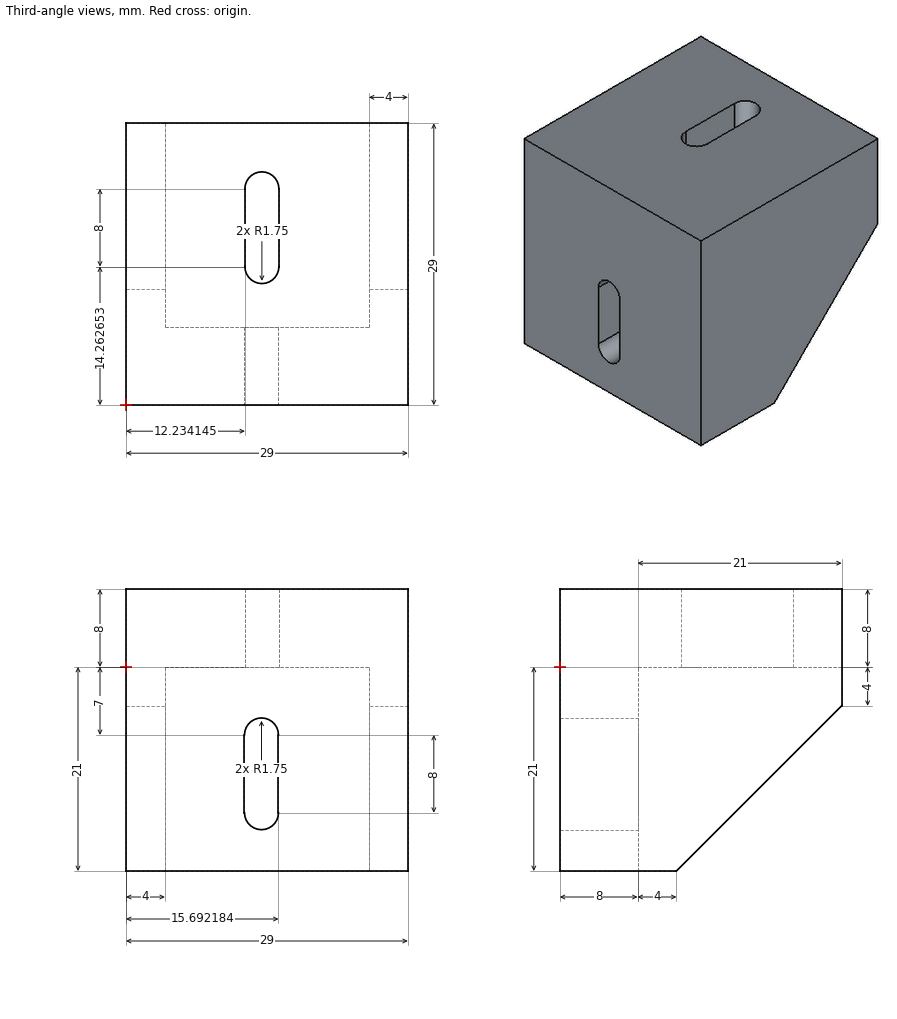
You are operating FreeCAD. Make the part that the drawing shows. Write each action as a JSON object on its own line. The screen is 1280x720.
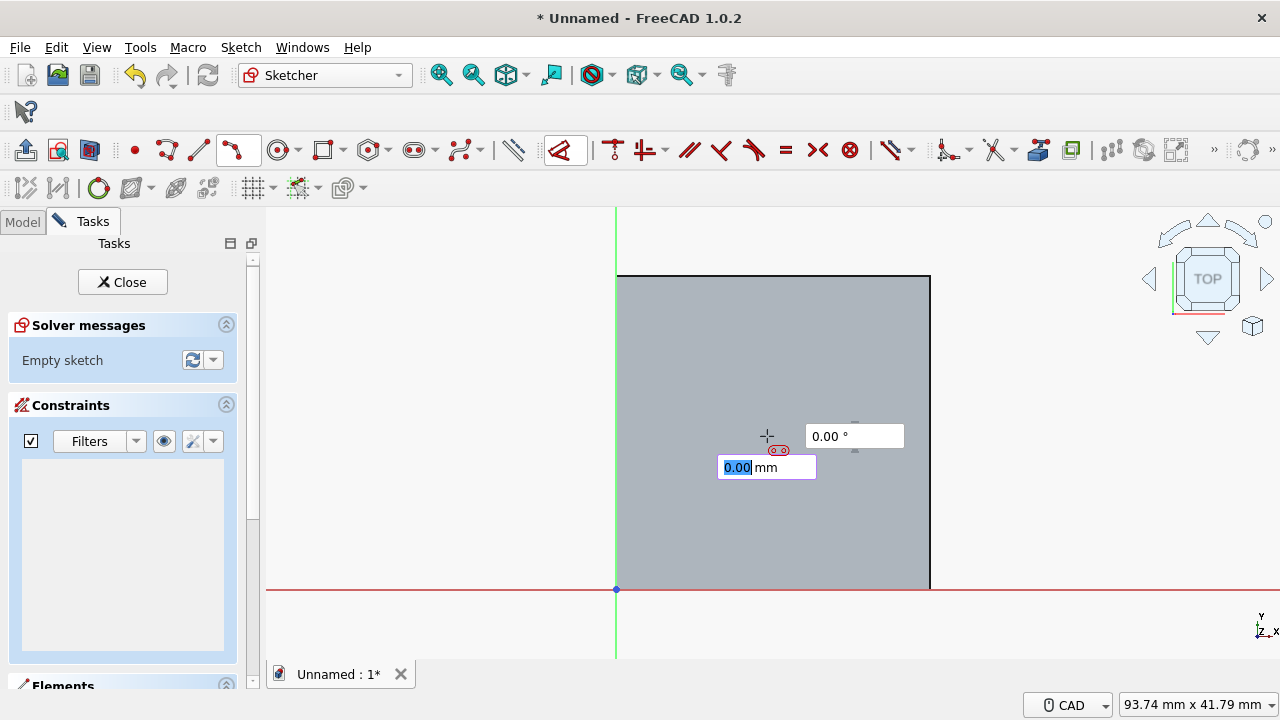
{"action": "left_click", "coordinate": [767, 349]}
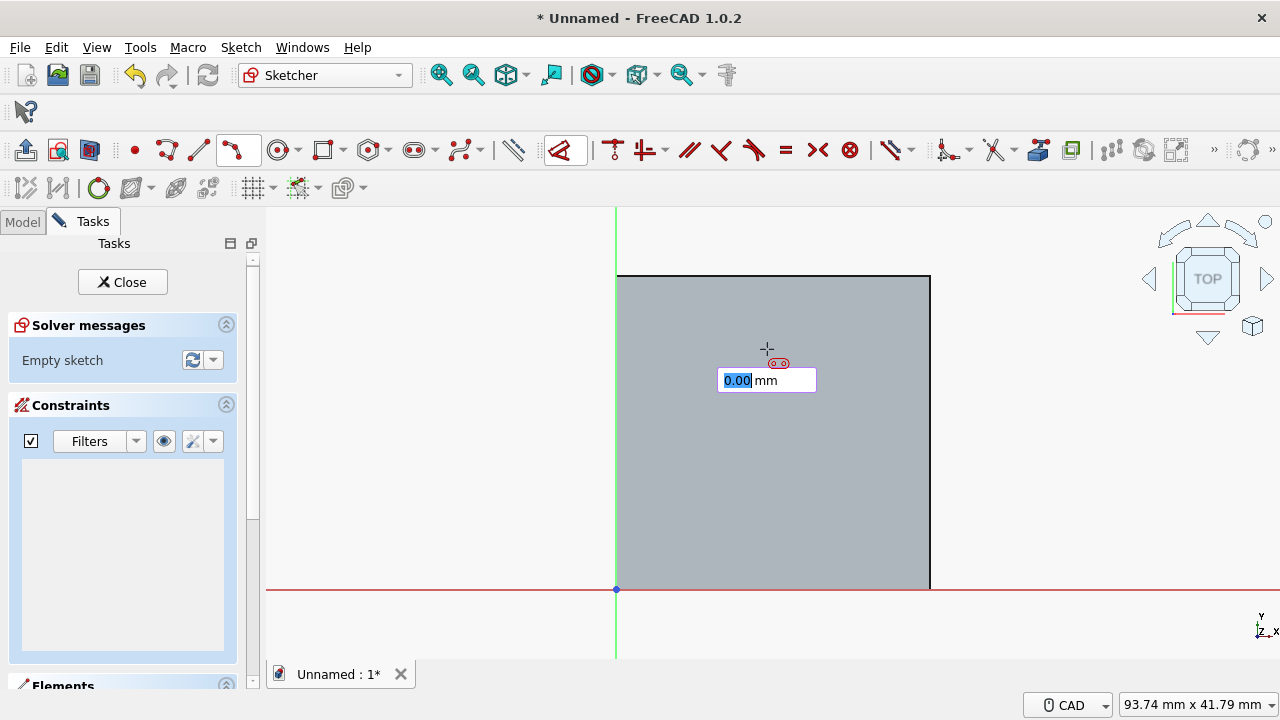
{"action": "left_click", "coordinate": [748, 392]}
{"action": "key", "text": "Escape"}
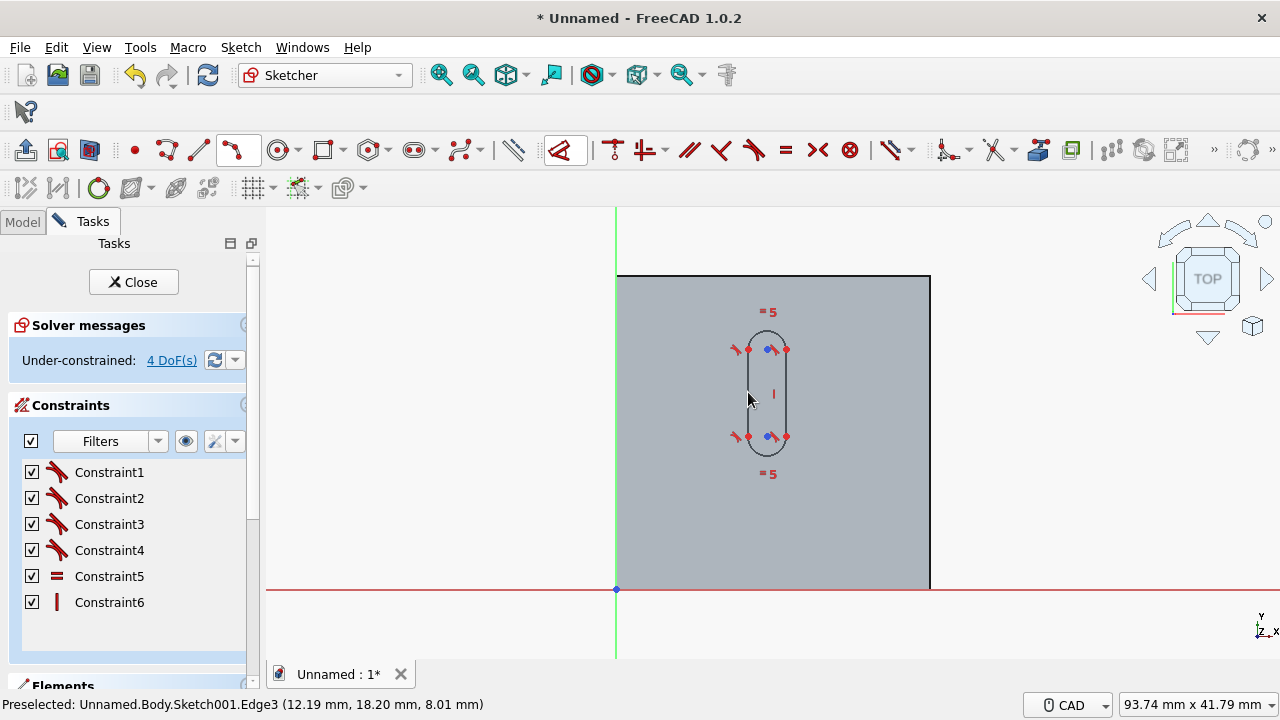
{"action": "scroll", "coordinate": [756, 452], "scroll_direction": "up", "scroll_amount": 4}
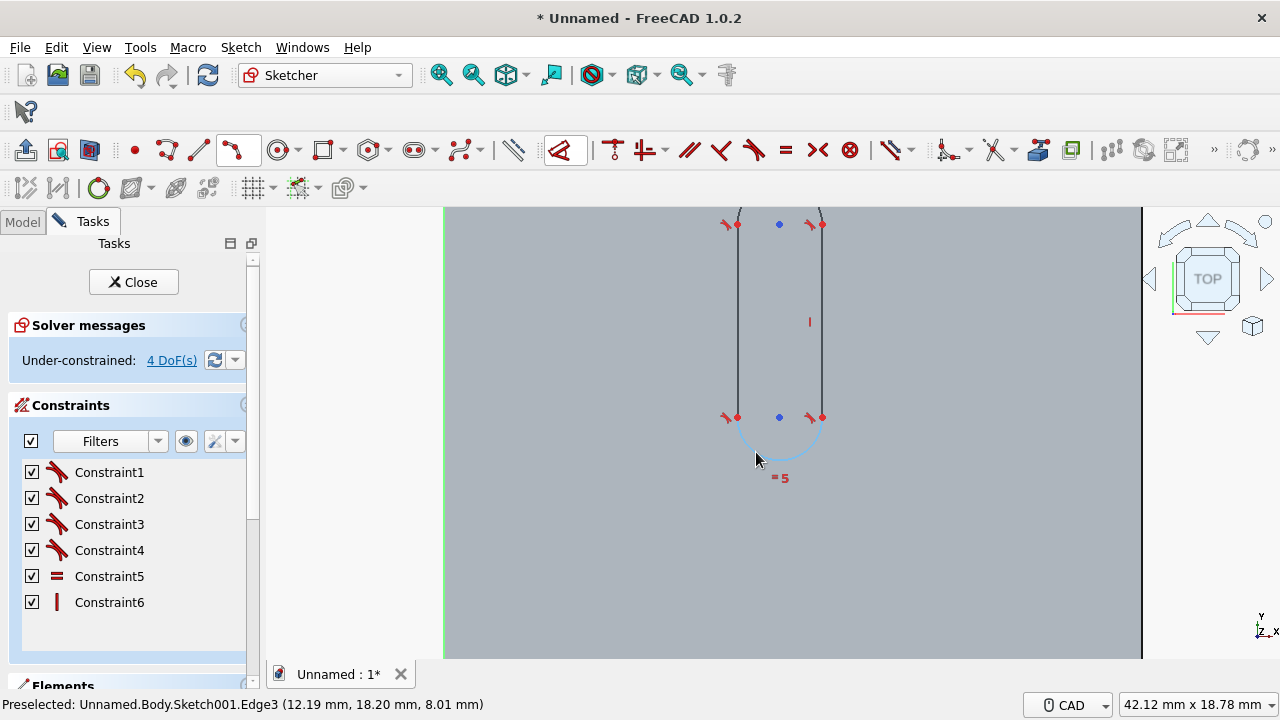
{"action": "left_click", "coordinate": [755, 452]}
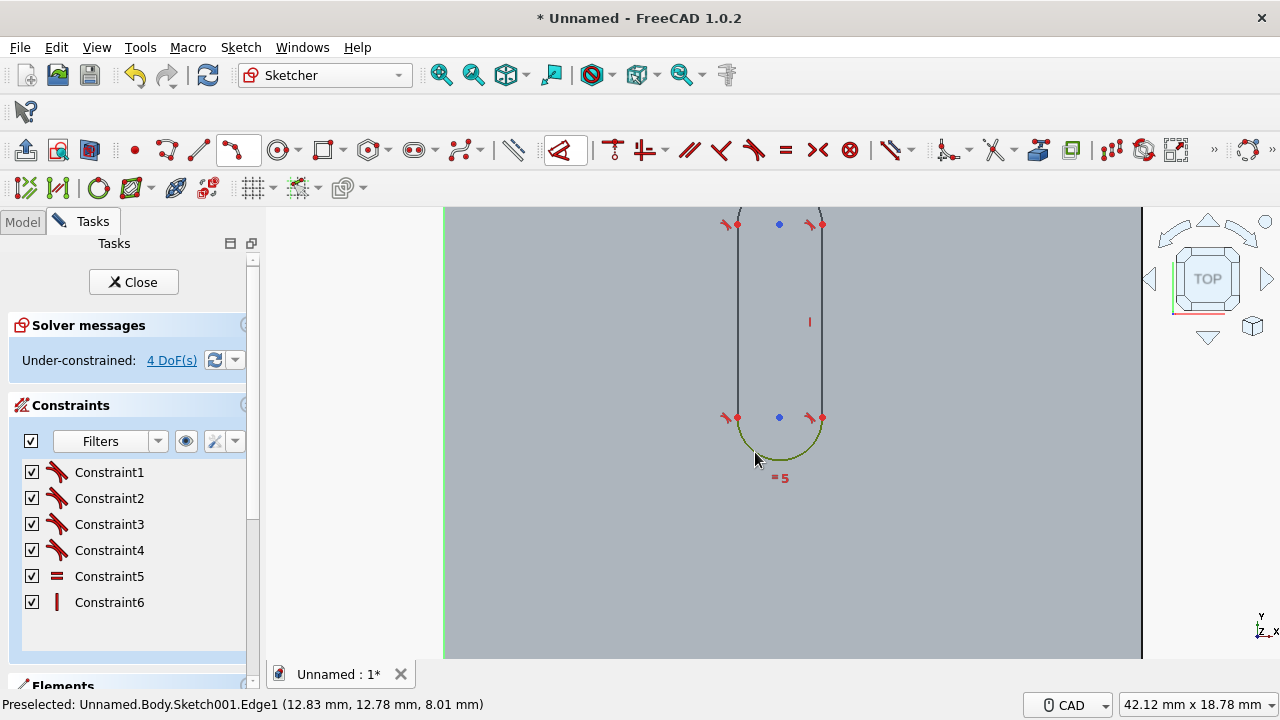
{"action": "left_click", "coordinate": [582, 150]}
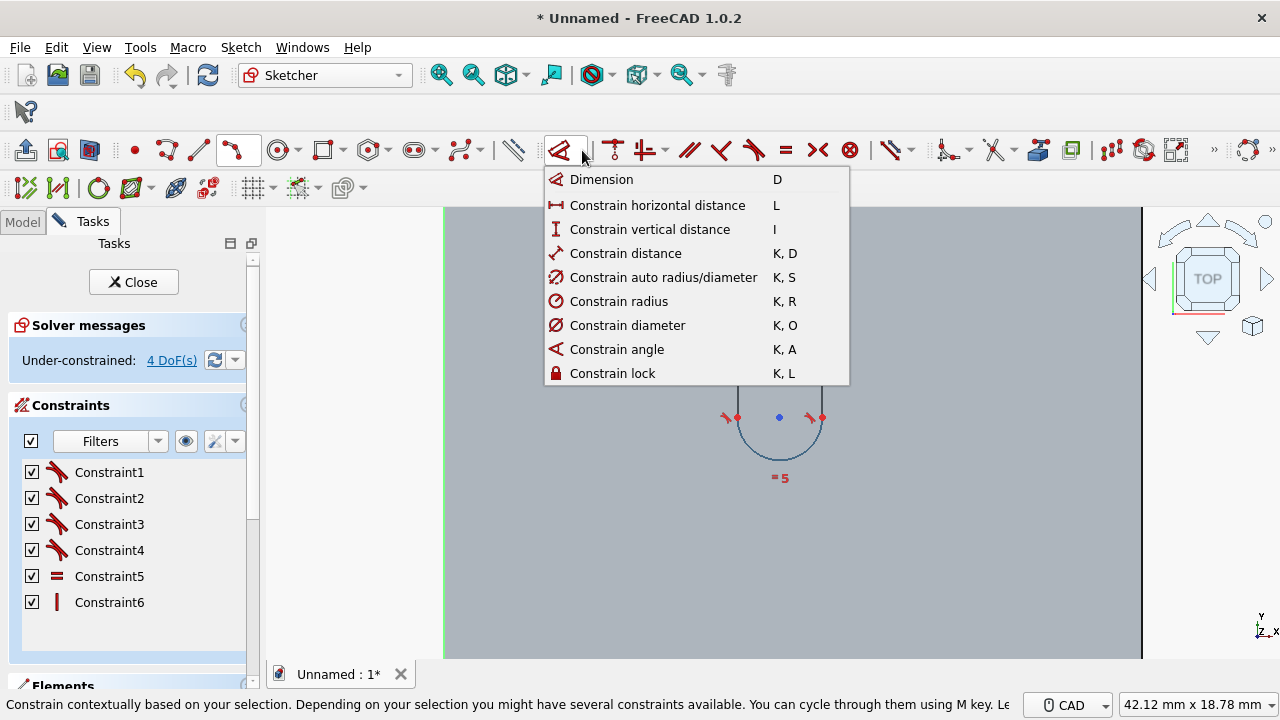
{"action": "left_click", "coordinate": [697, 301]}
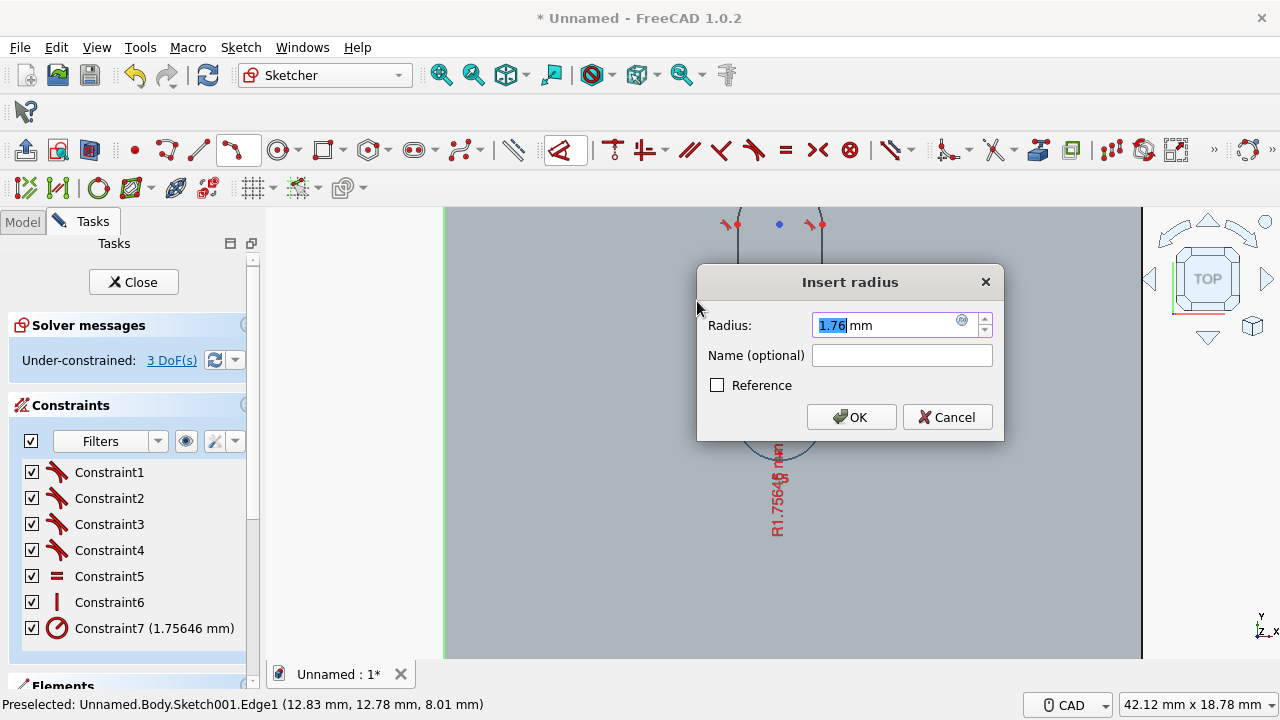
{"action": "type", "text": "1.75"}
{"action": "key", "text": "Return"}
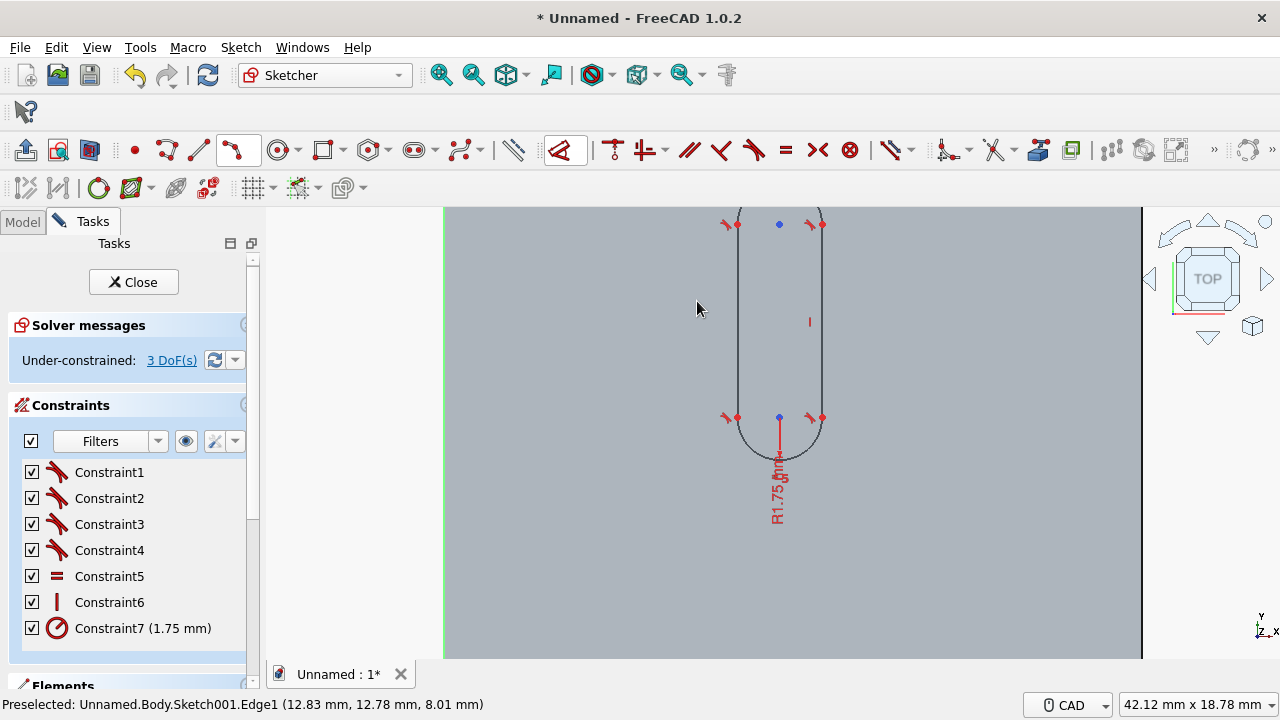
{"action": "left_click", "coordinate": [738, 360]}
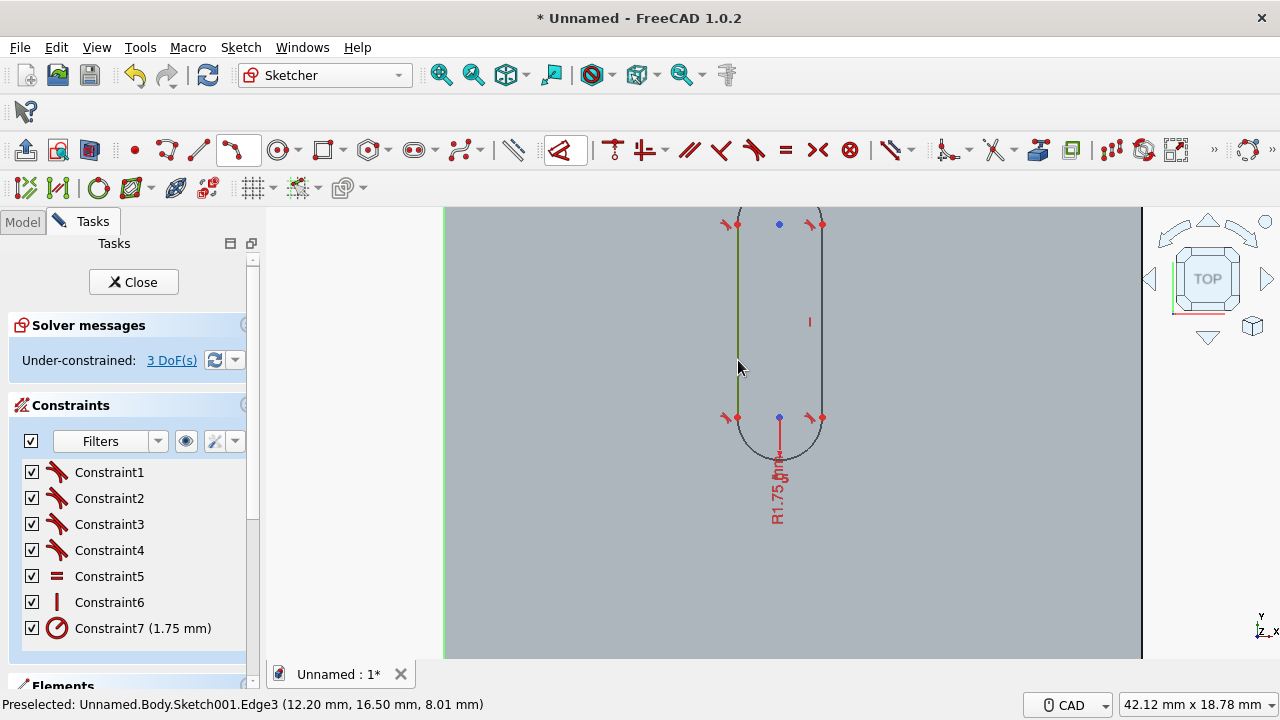
{"action": "left_click", "coordinate": [582, 150]}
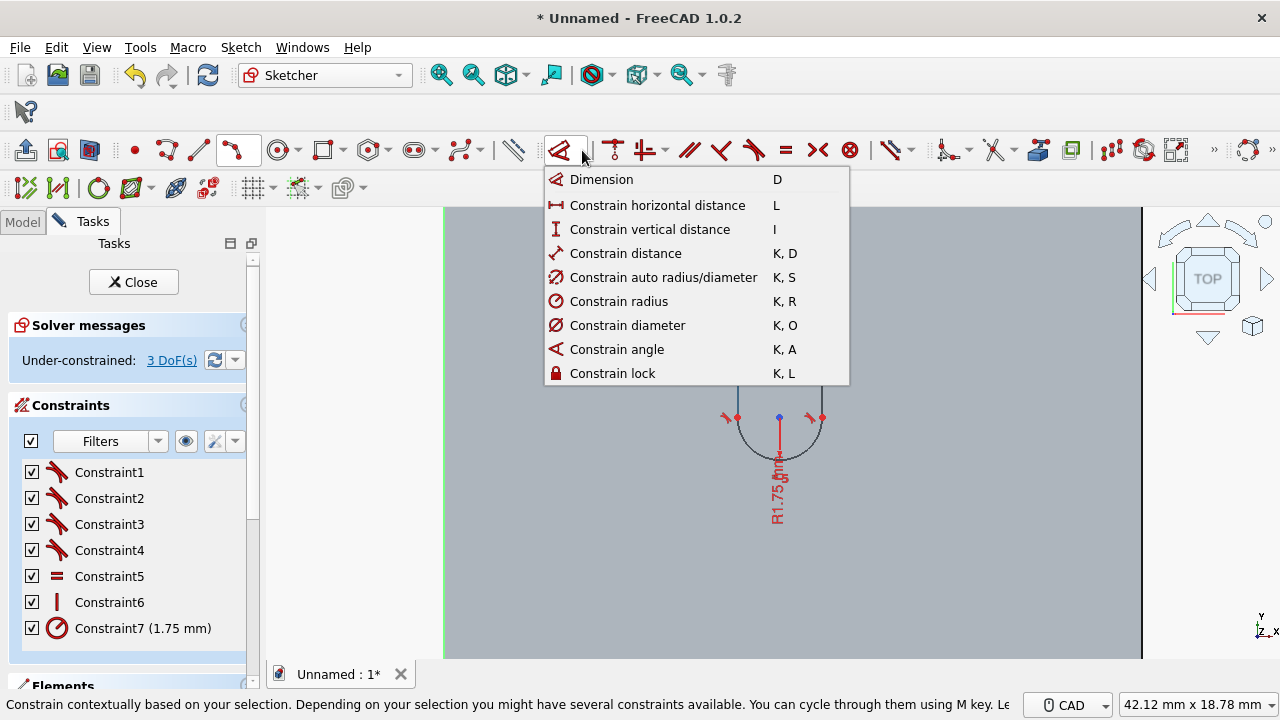
{"action": "left_click", "coordinate": [697, 229]}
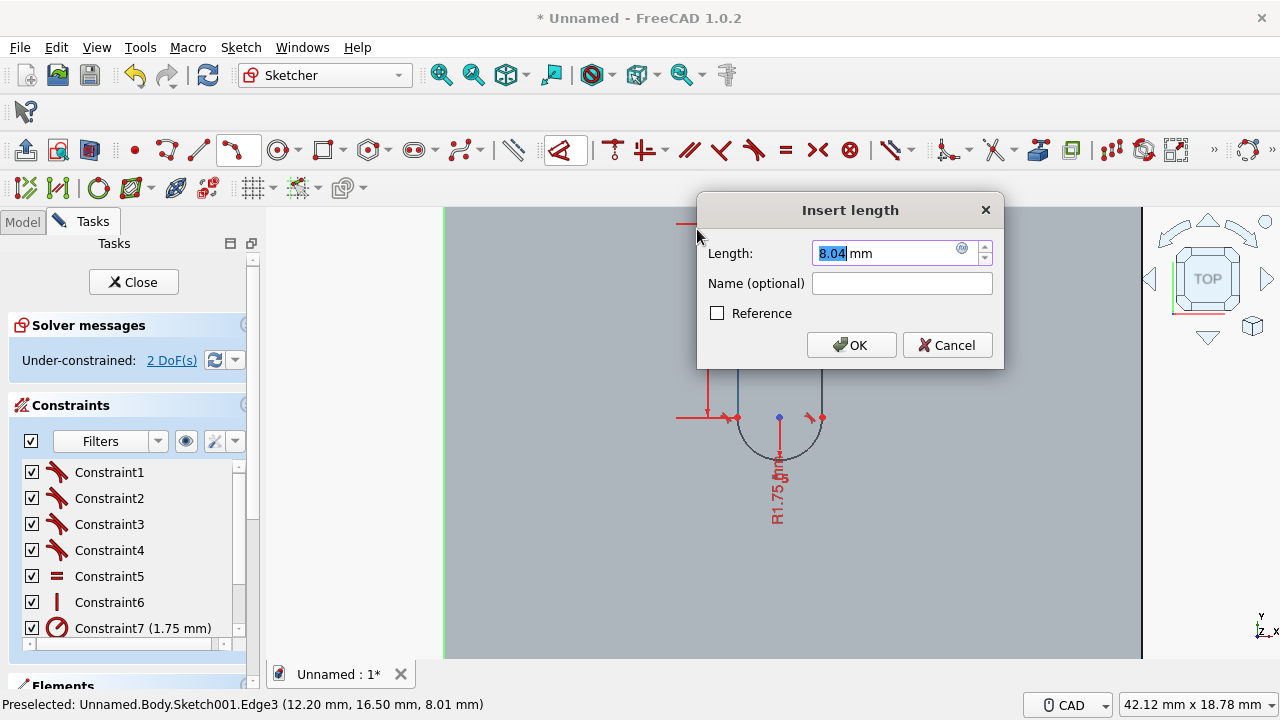
{"action": "type", "text": "8"}
{"action": "key", "text": "Return"}